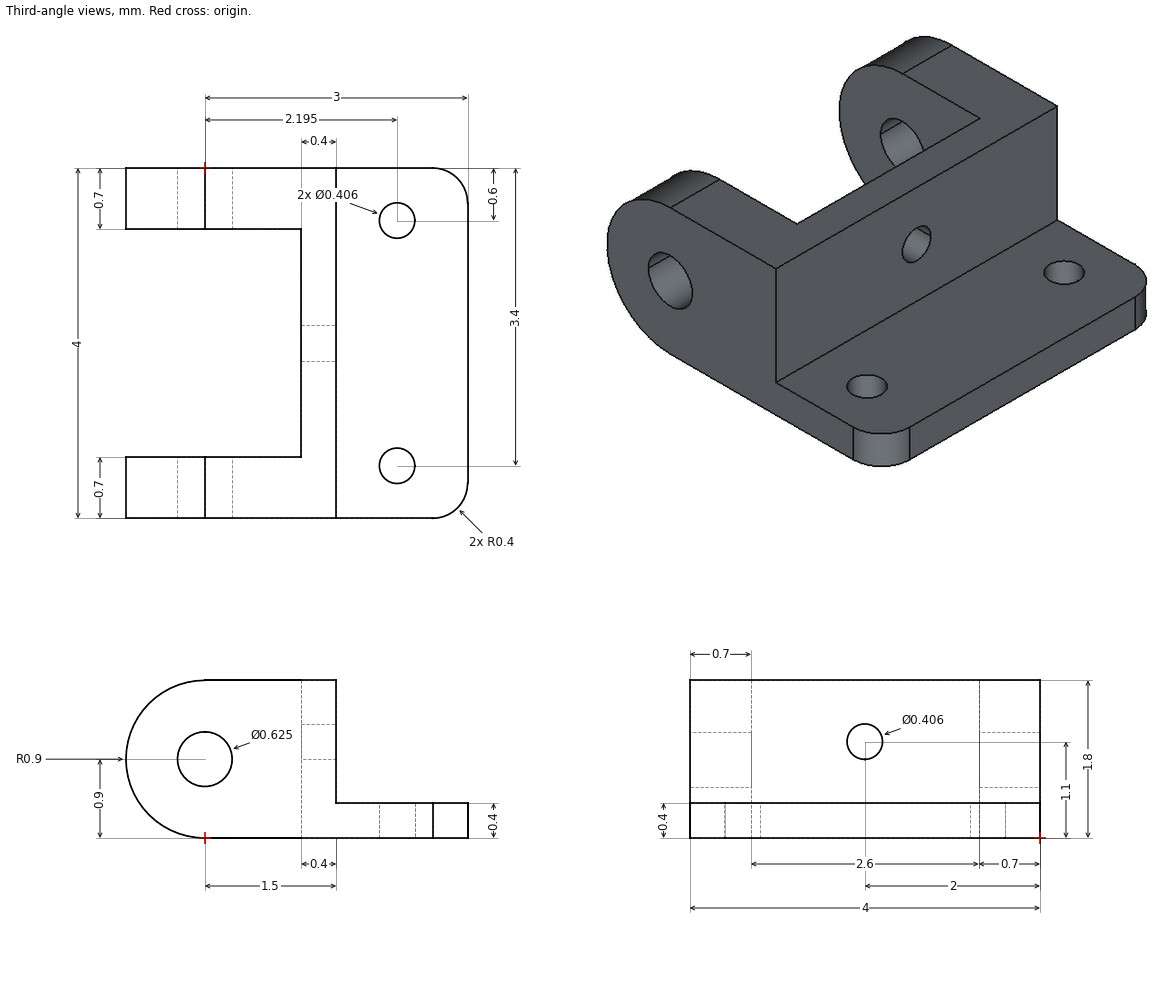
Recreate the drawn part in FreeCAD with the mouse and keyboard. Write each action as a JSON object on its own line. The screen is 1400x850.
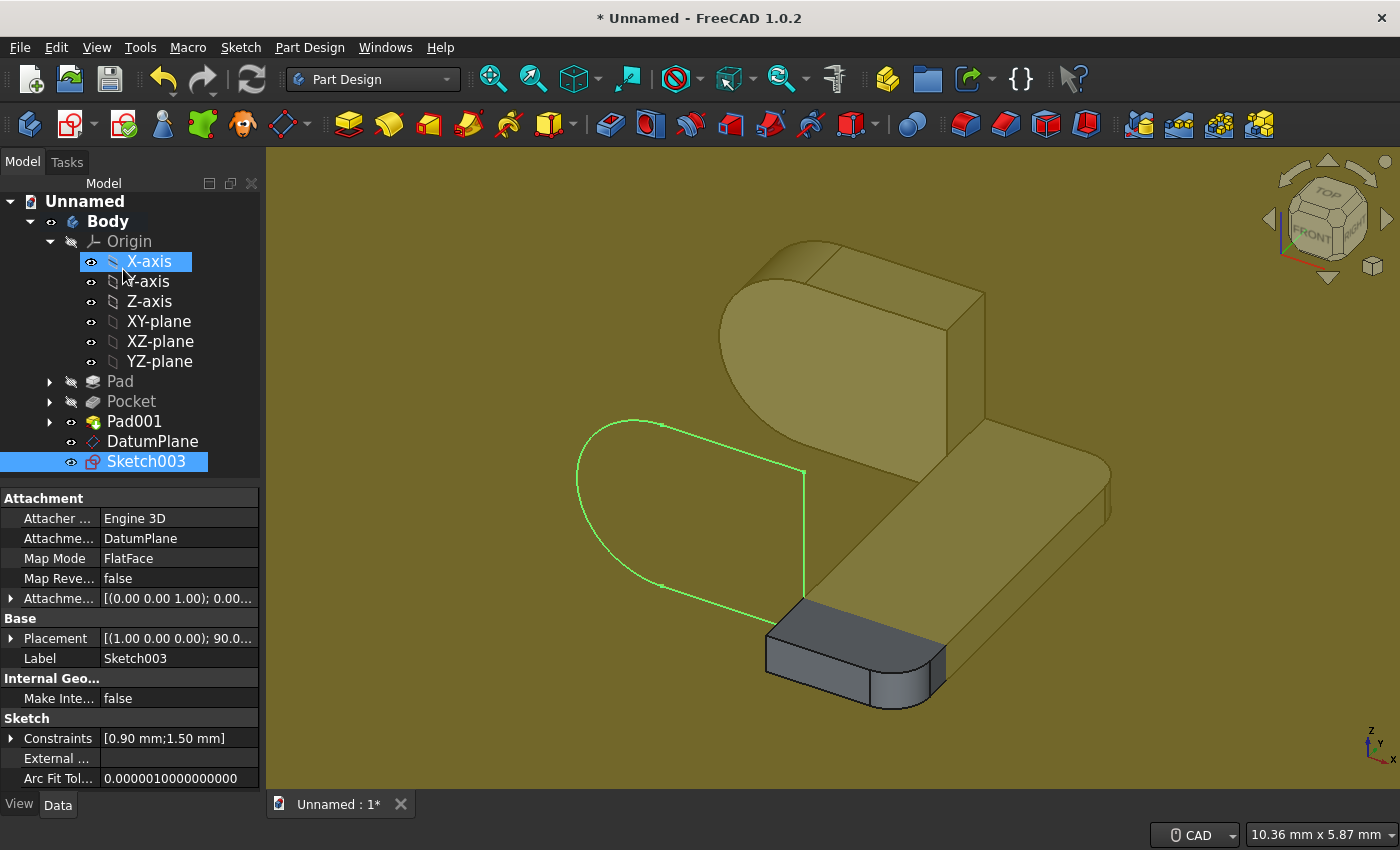
{"action": "left_click", "coordinate": [350, 124]}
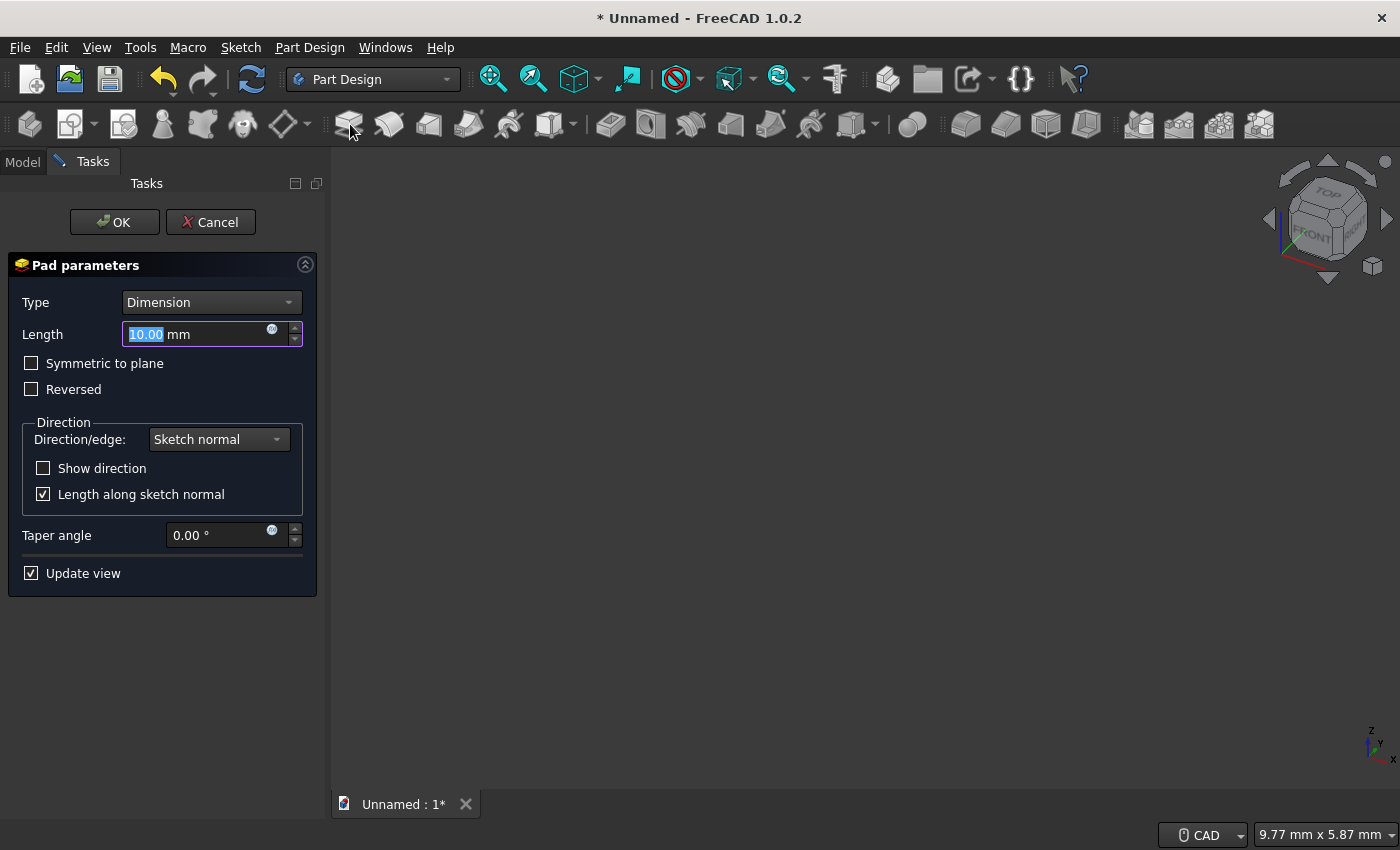
{"action": "type", "text": "0.7"}
{"action": "key", "text": "Tab"}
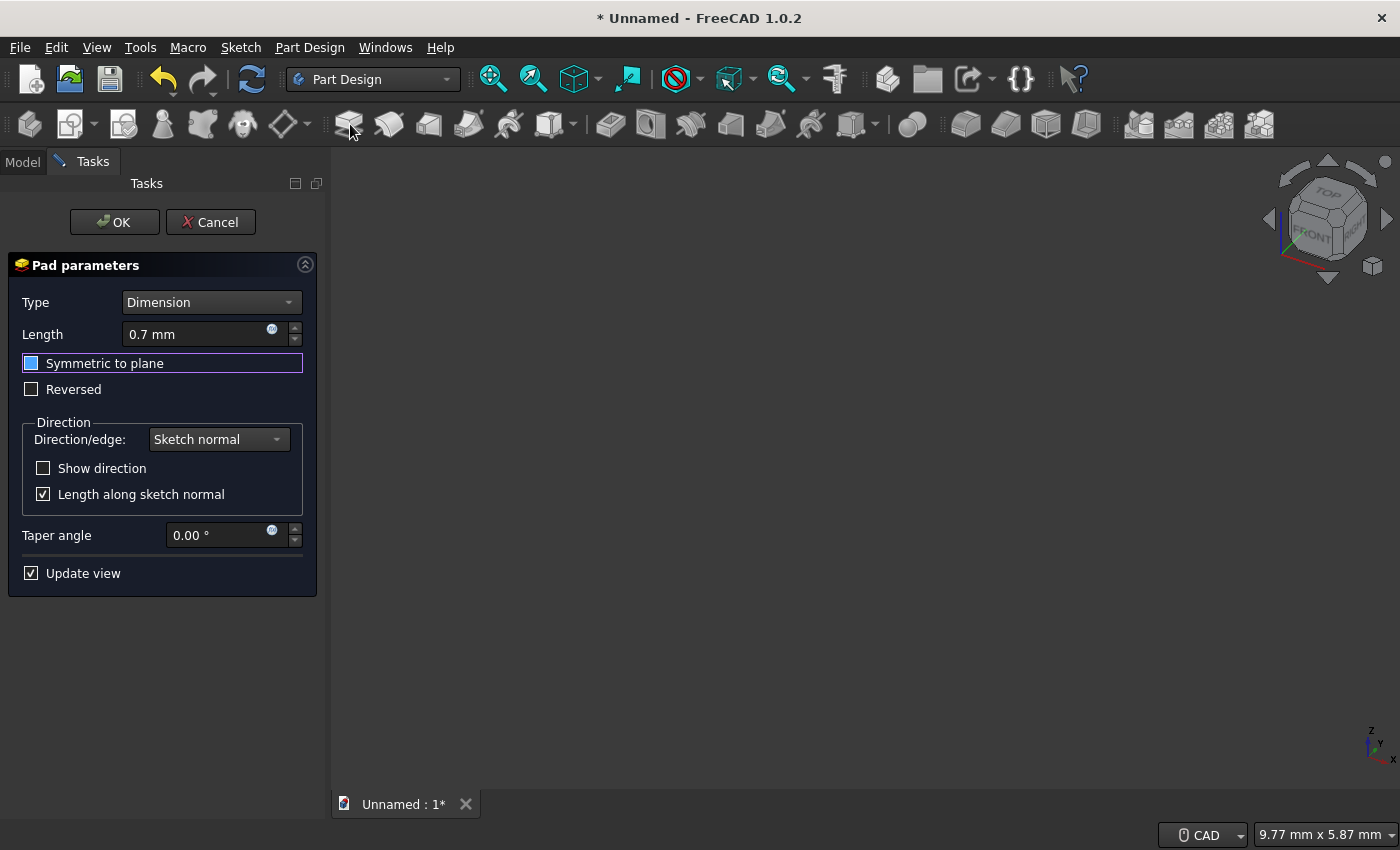
{"action": "left_click", "coordinate": [115, 222]}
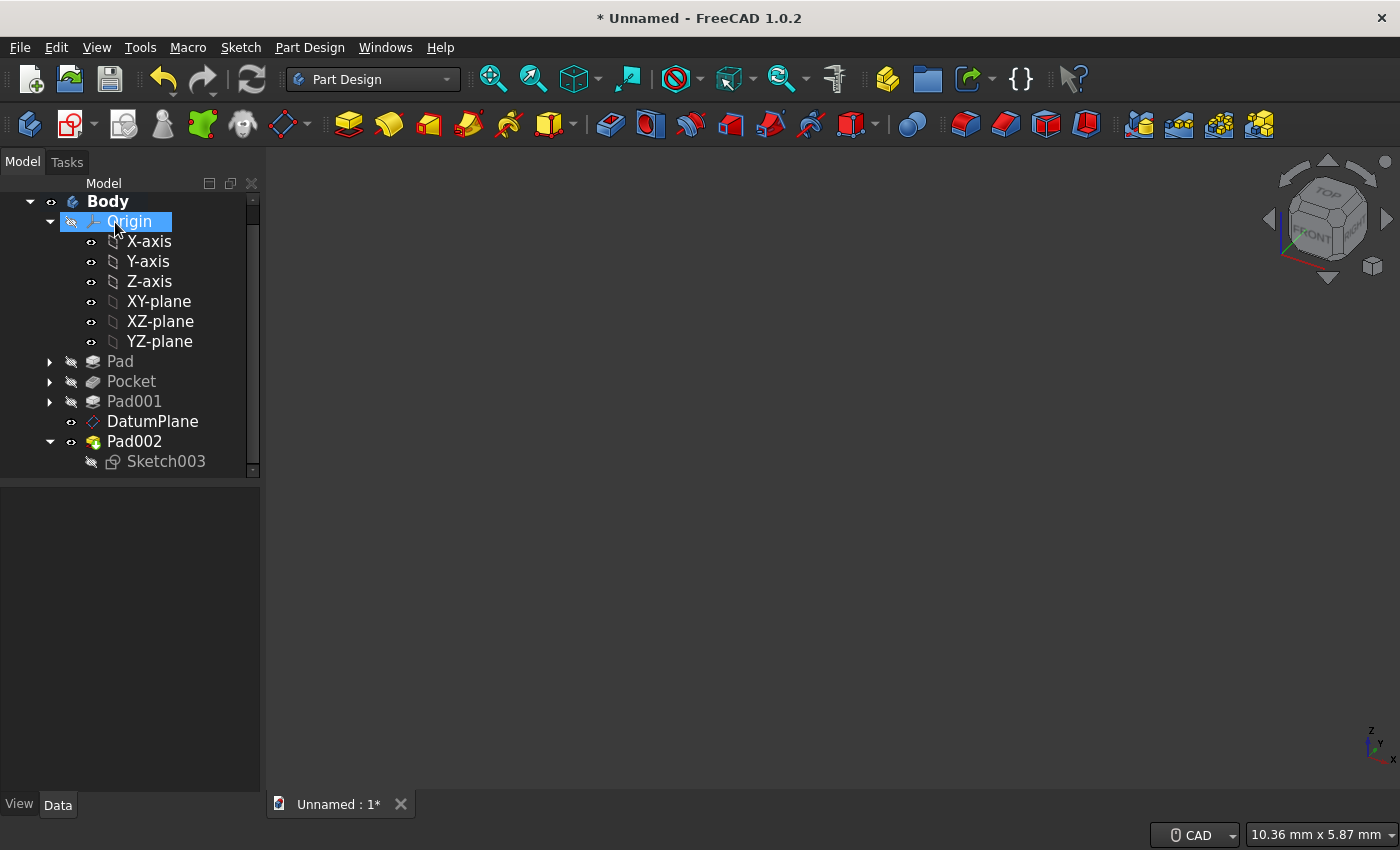
{"action": "left_click", "coordinate": [116, 422]}
{"action": "key", "text": "space"}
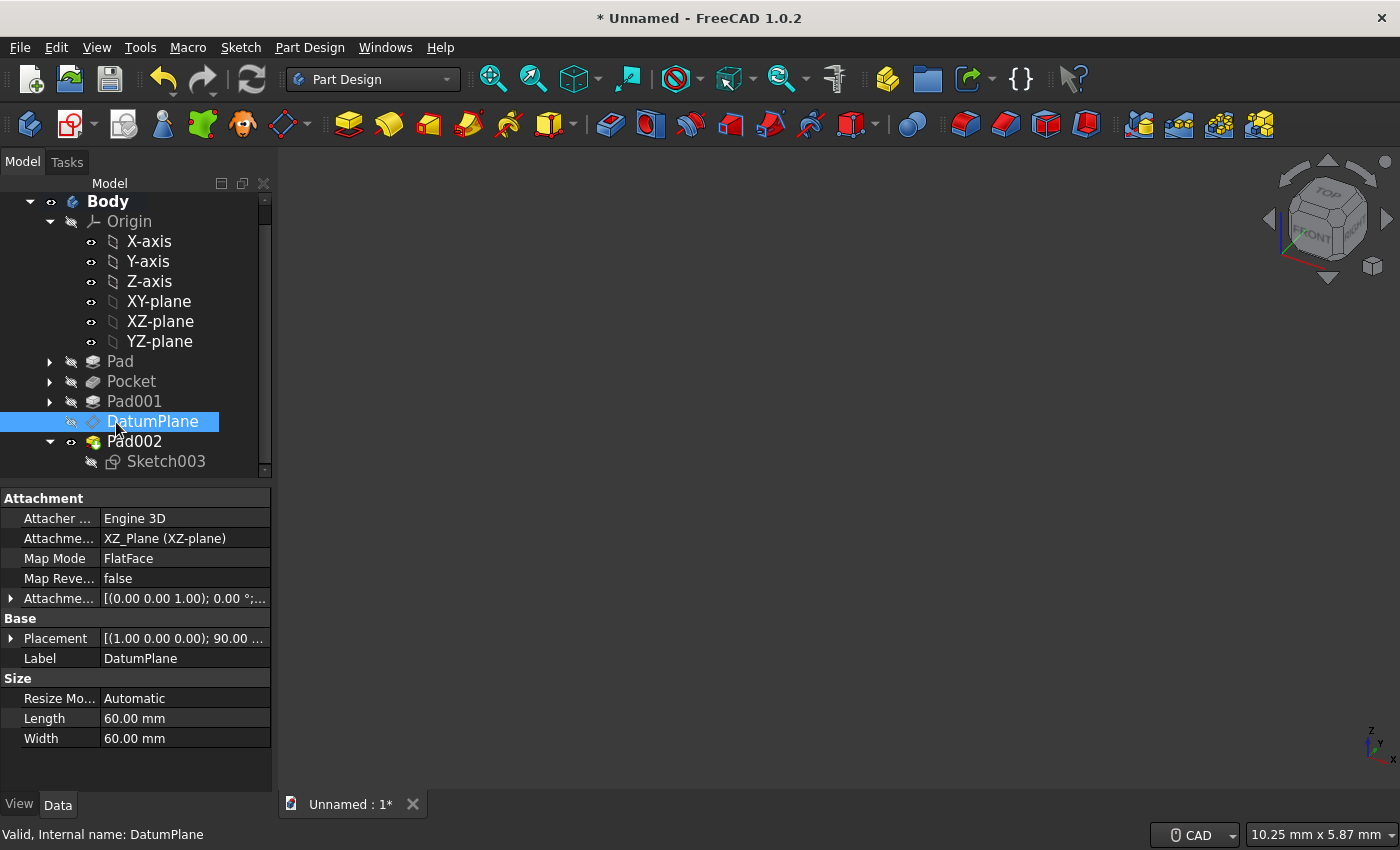
{"action": "key", "text": "v f"}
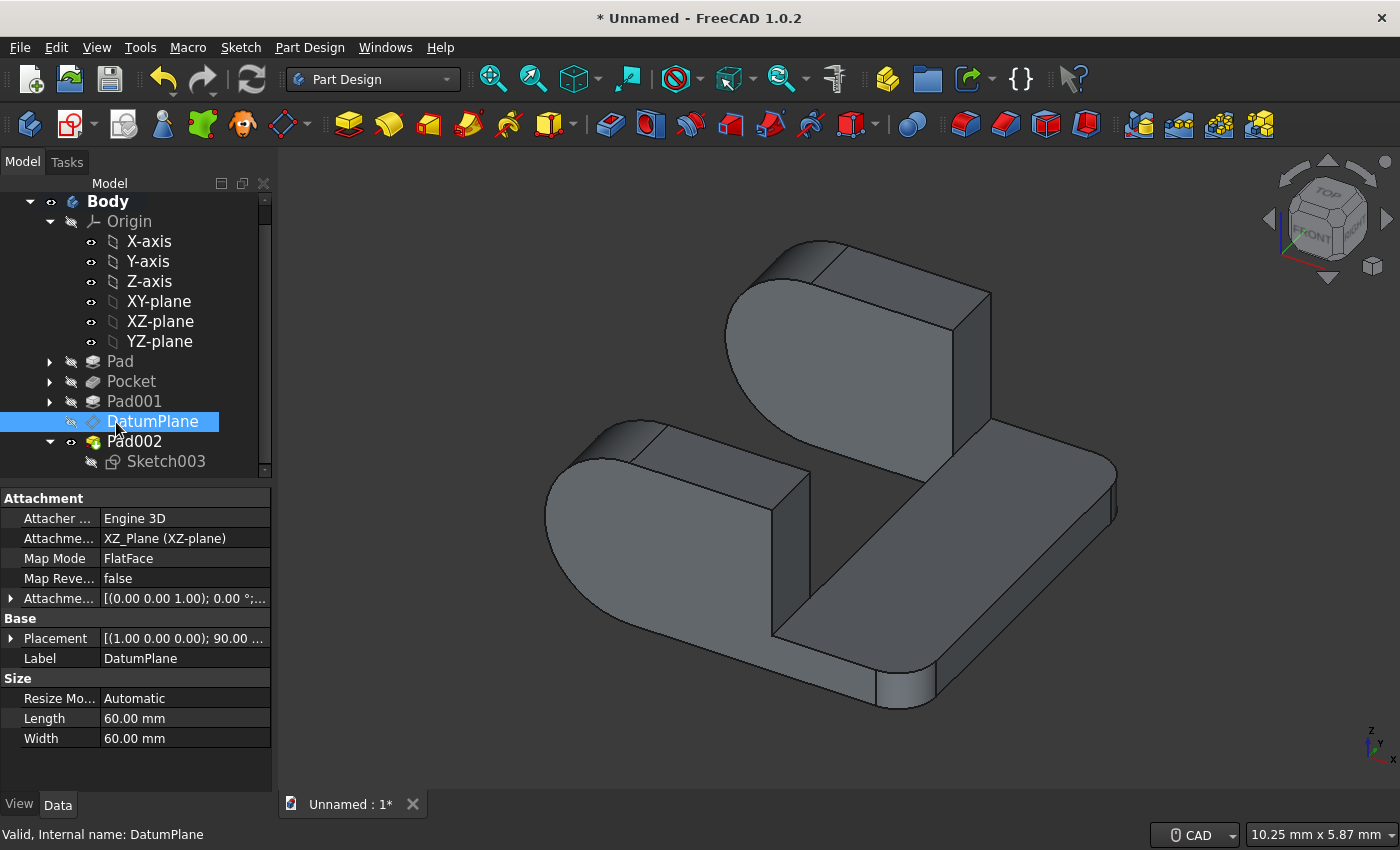
{"action": "key", "text": "6"}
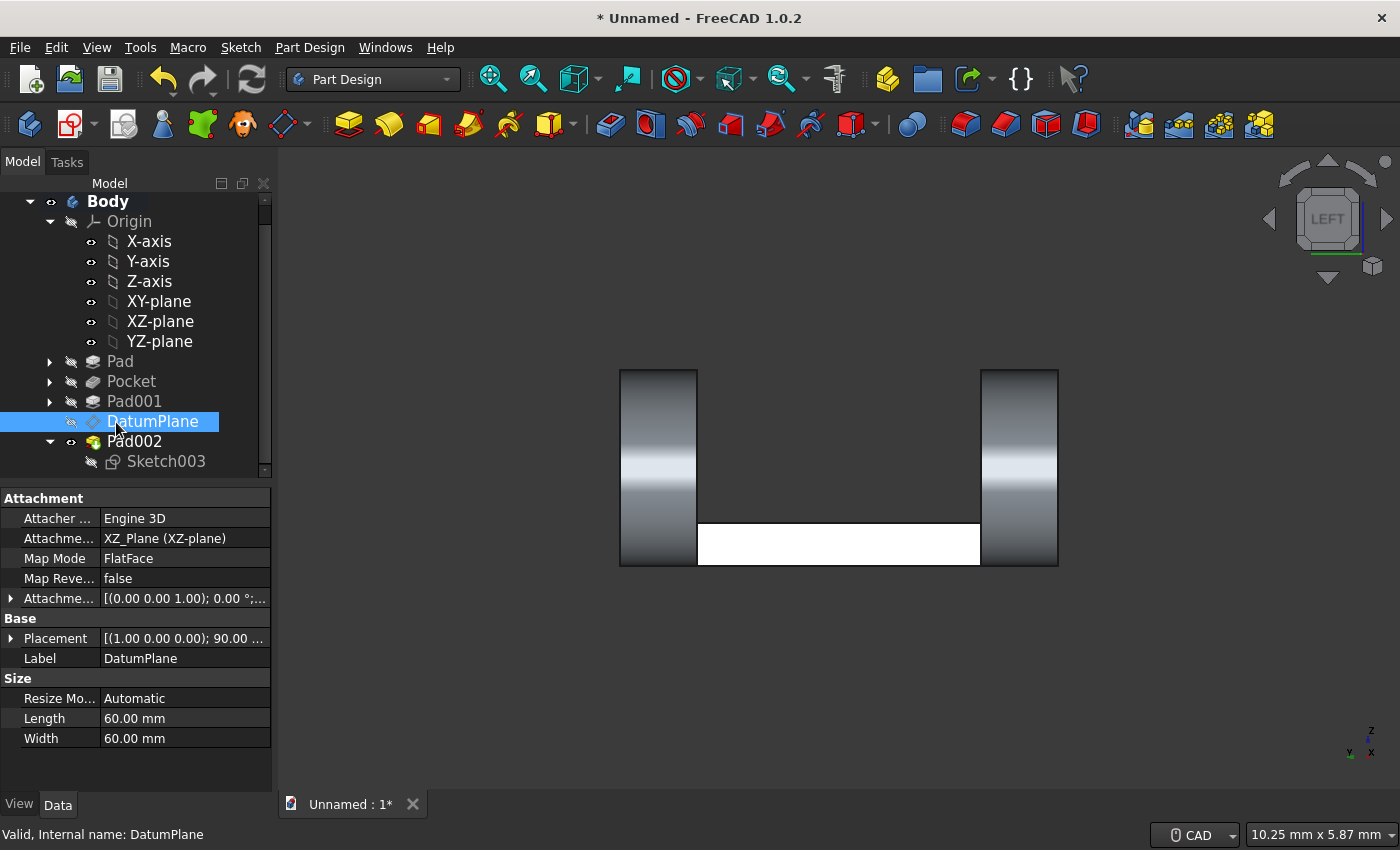
{"action": "left_click", "coordinate": [494, 80]}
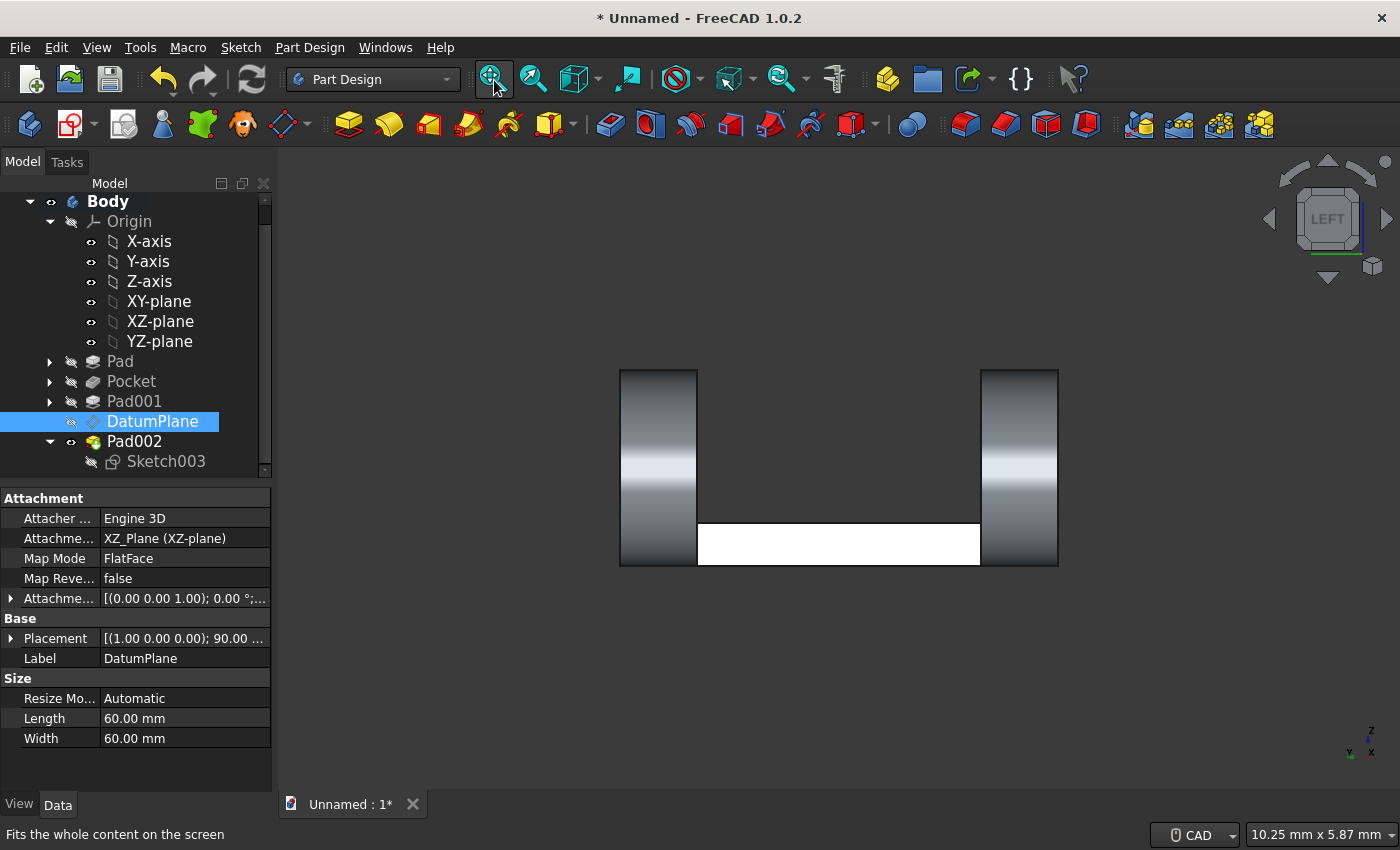
{"action": "left_click", "coordinate": [758, 544]}